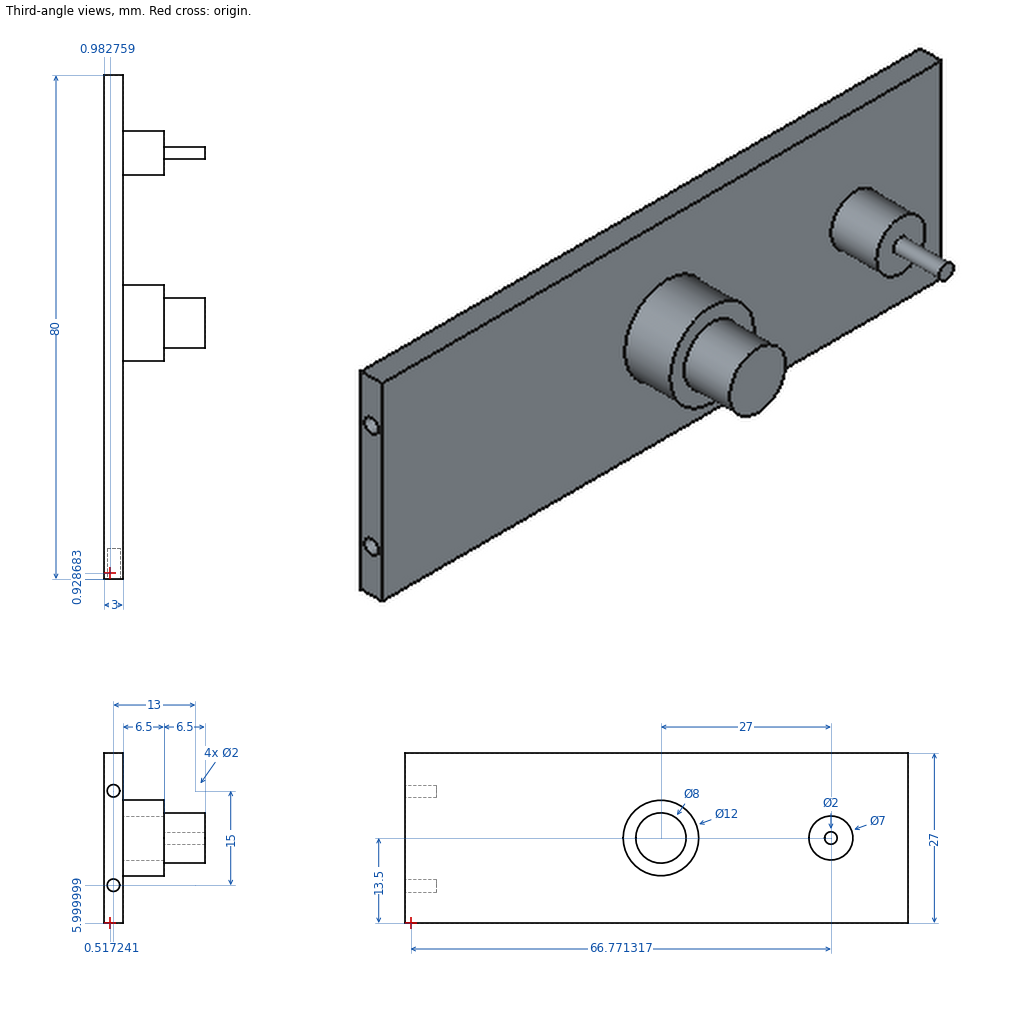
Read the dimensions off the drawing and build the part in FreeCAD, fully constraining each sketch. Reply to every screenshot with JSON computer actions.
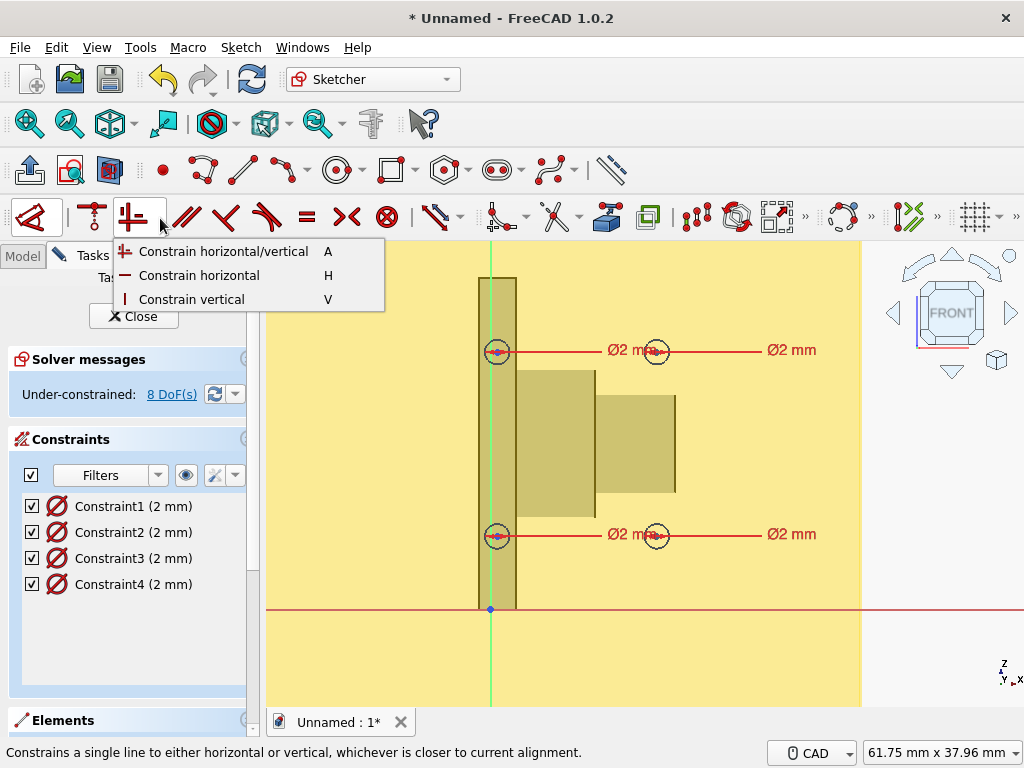
{"action": "left_click", "coordinate": [249, 299]}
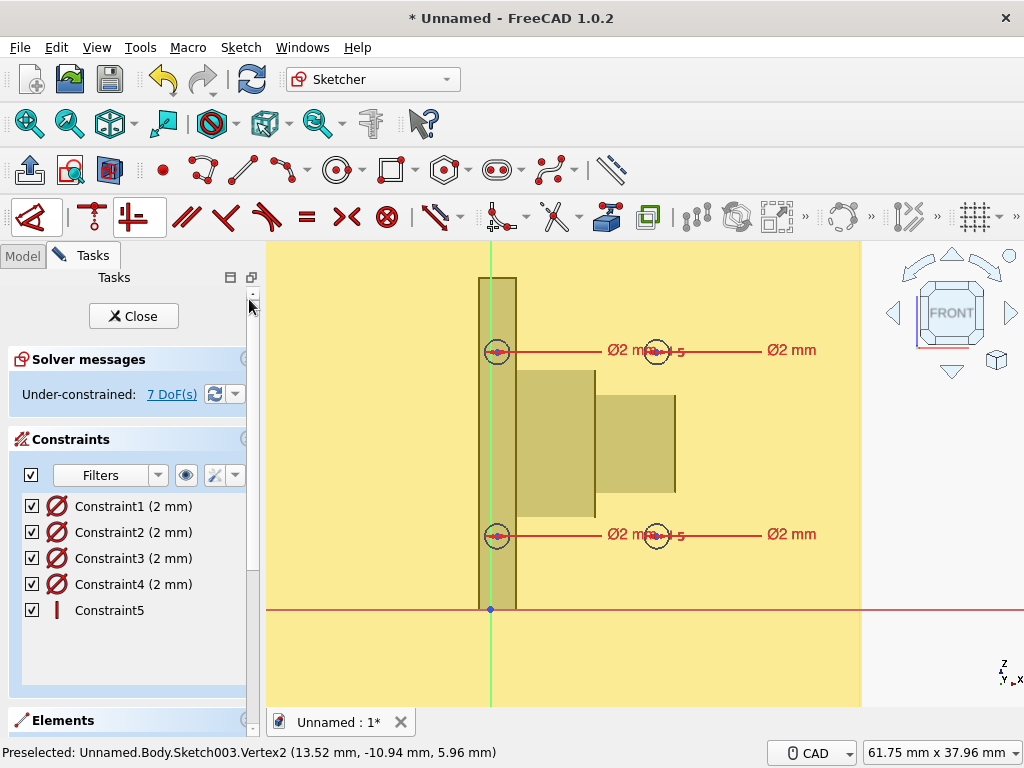
{"action": "left_click", "coordinate": [657, 352]}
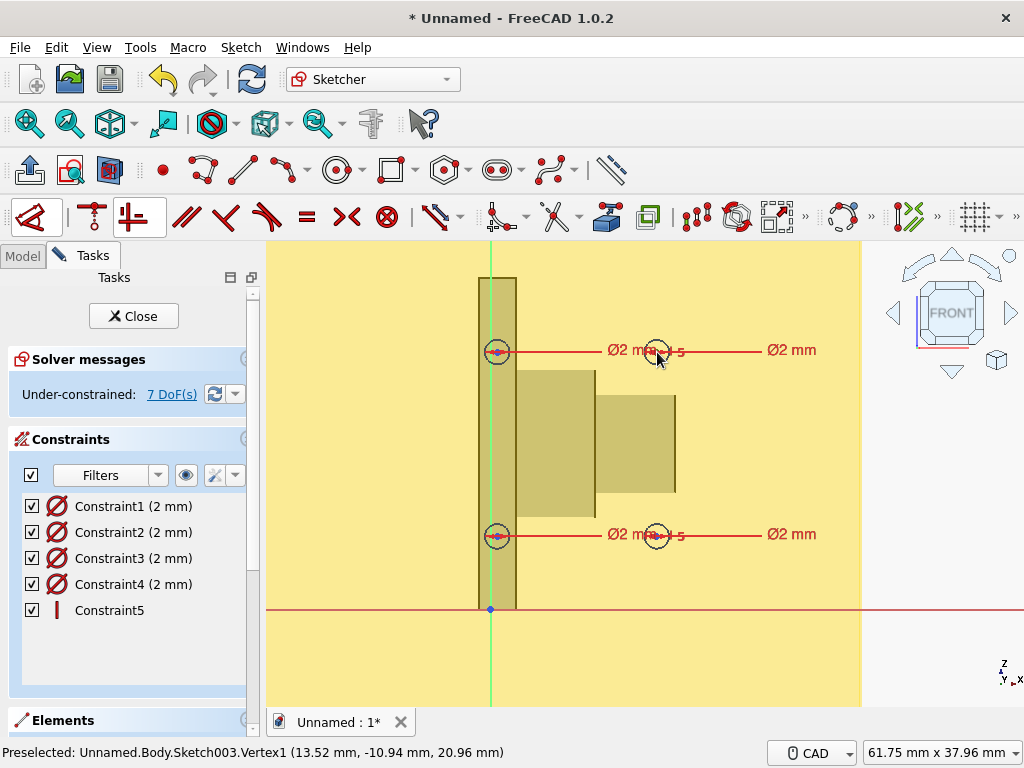
{"action": "left_click", "coordinate": [497, 352]}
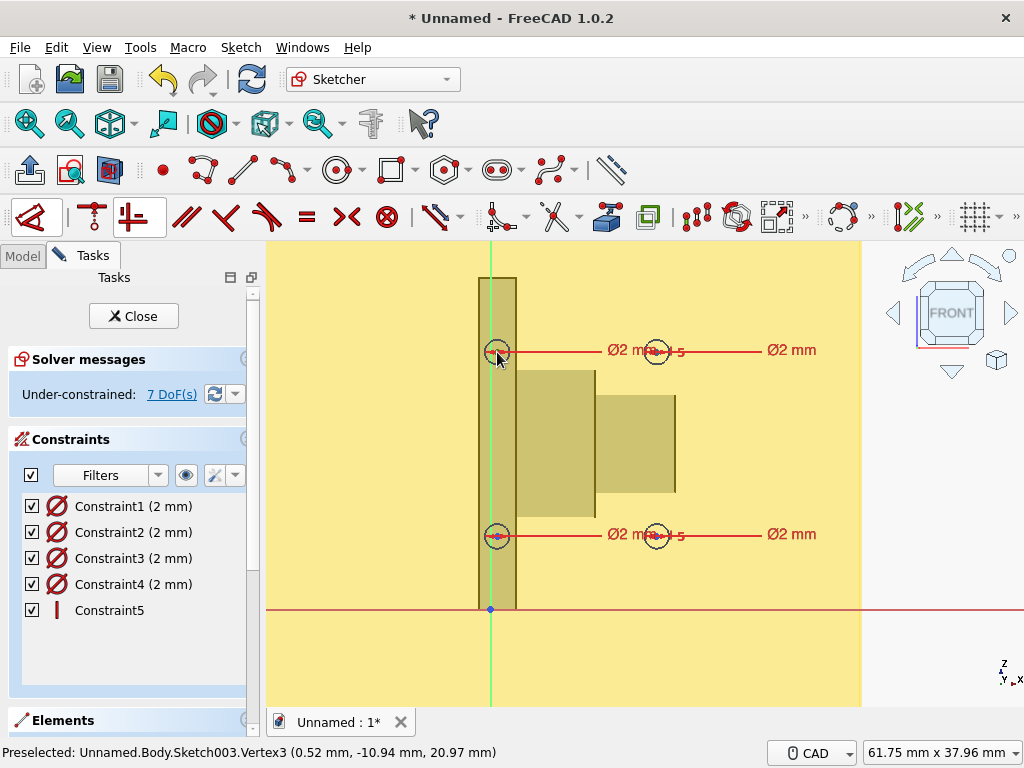
{"action": "left_click", "coordinate": [160, 218]}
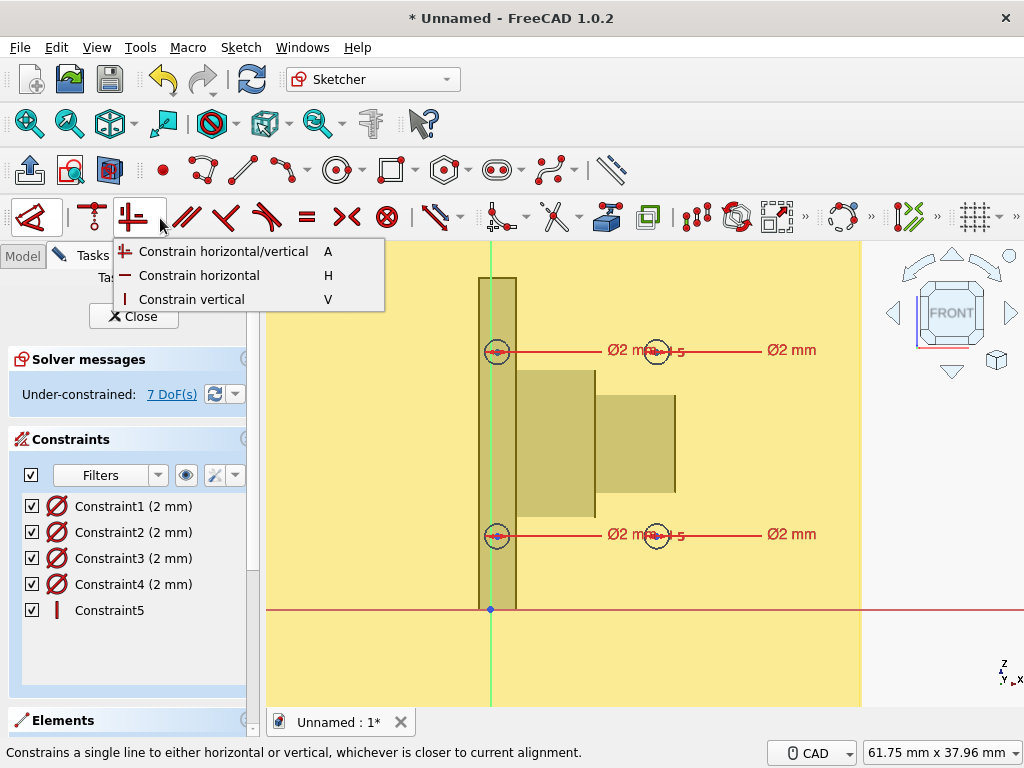
{"action": "left_click", "coordinate": [249, 275]}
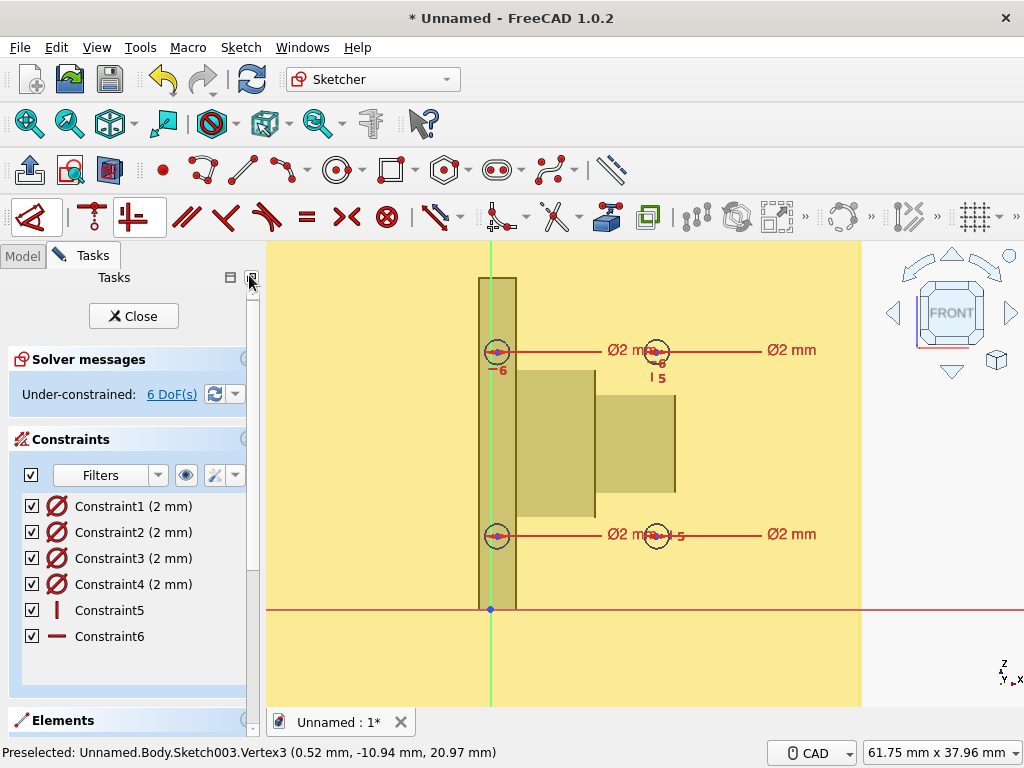
{"action": "left_click", "coordinate": [497, 352]}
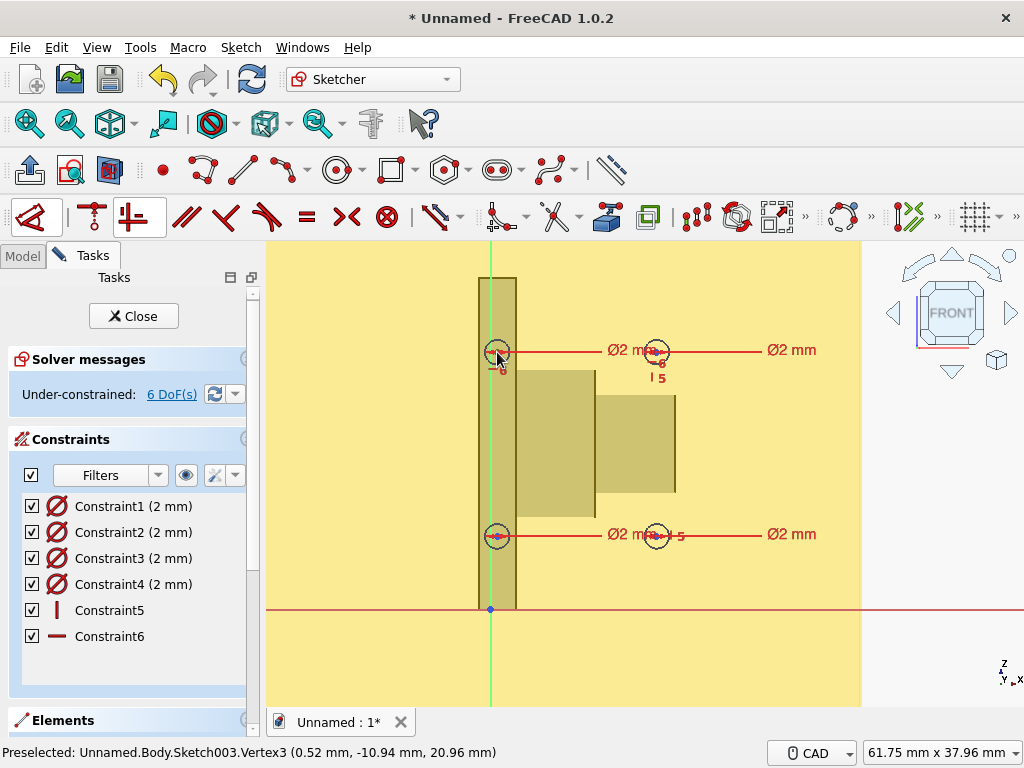
{"action": "left_click", "coordinate": [497, 536]}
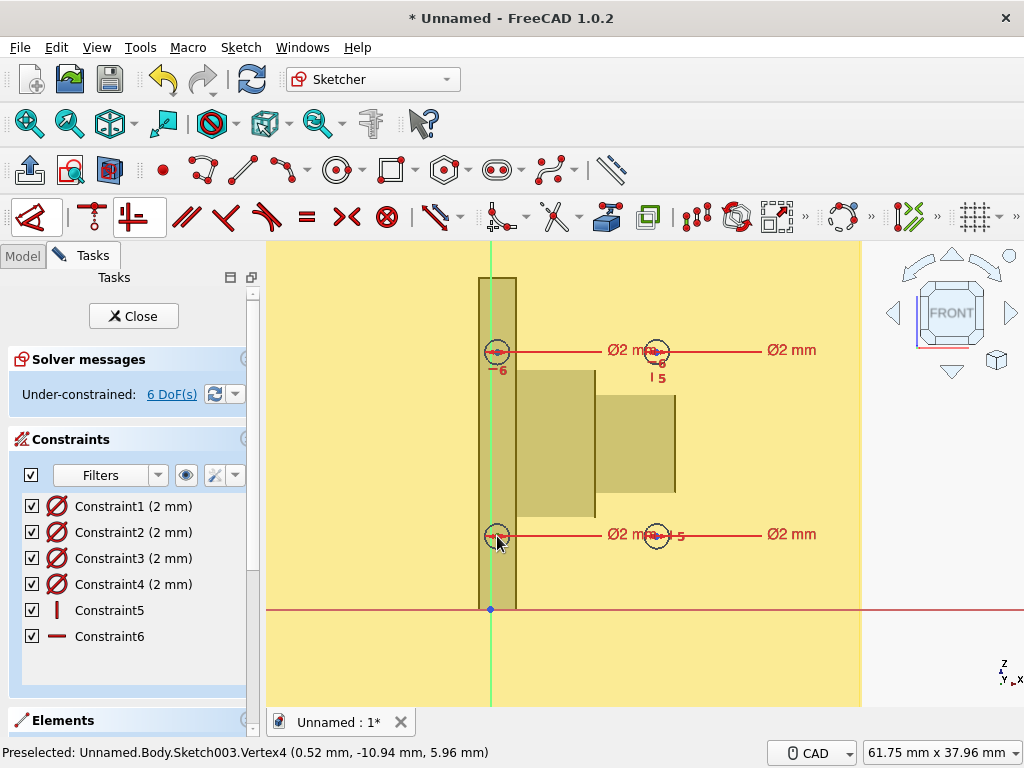
{"action": "left_click", "coordinate": [160, 218]}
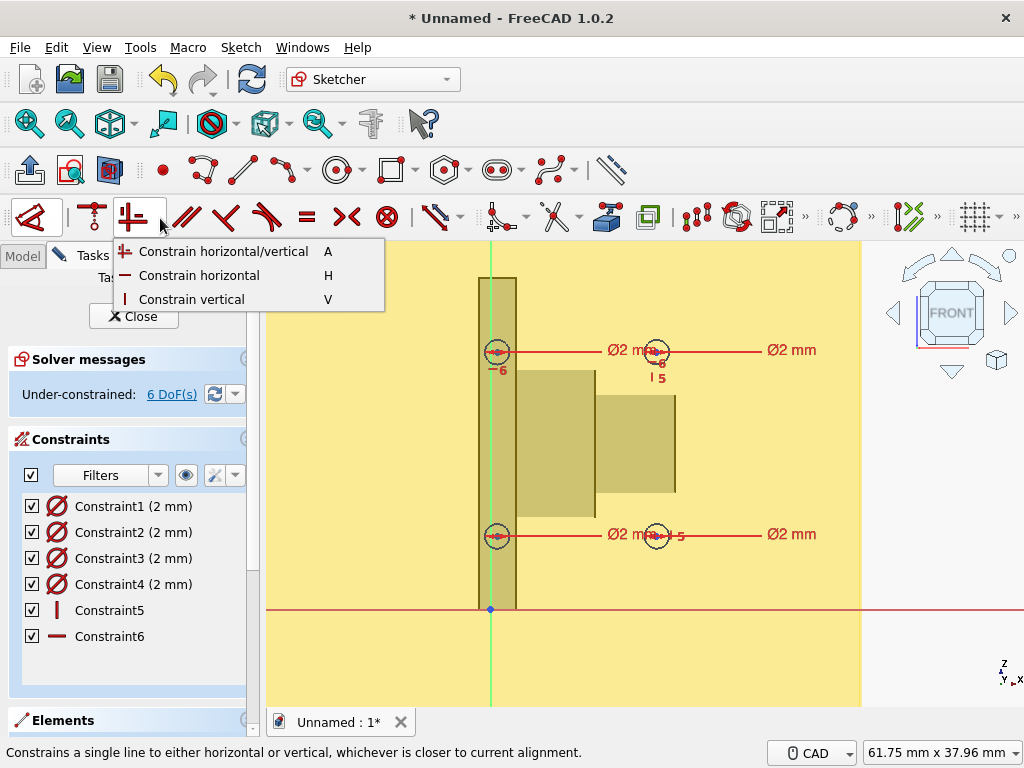
{"action": "left_click", "coordinate": [249, 299]}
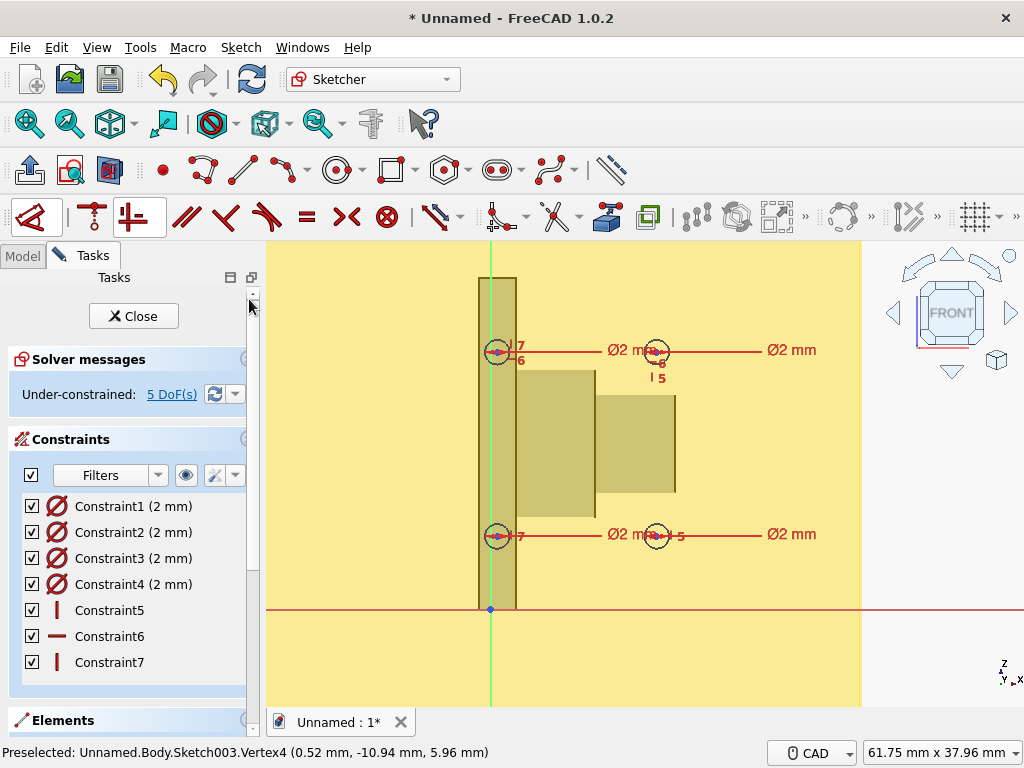
{"action": "left_click", "coordinate": [657, 536]}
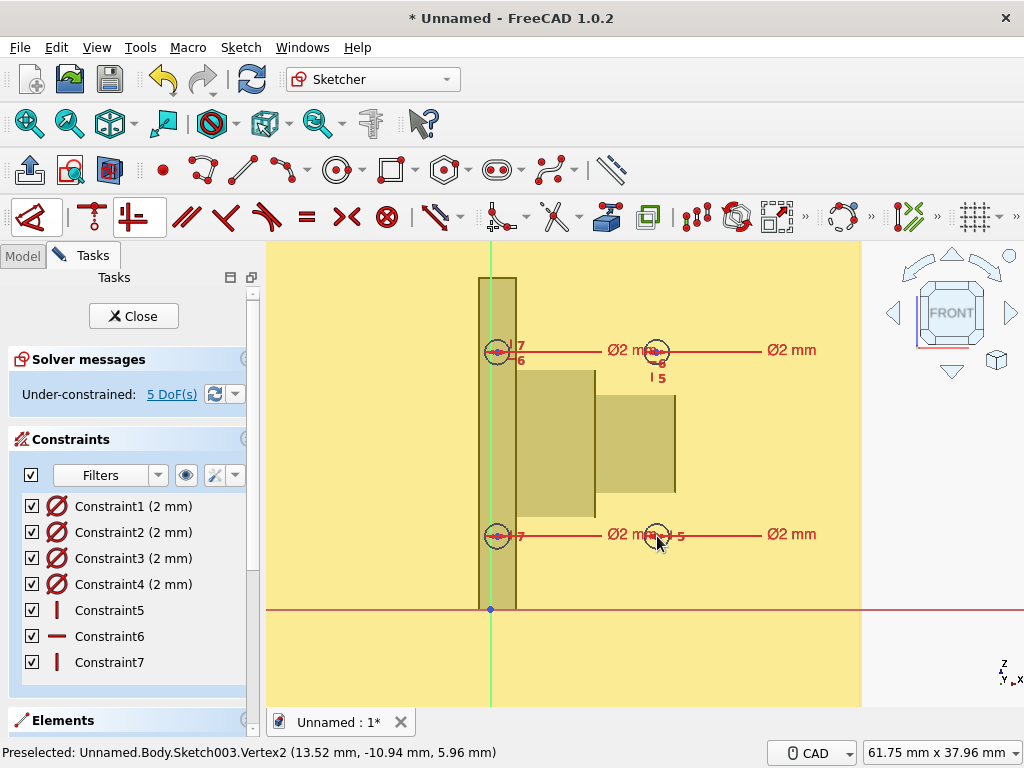
{"action": "left_click", "coordinate": [497, 536]}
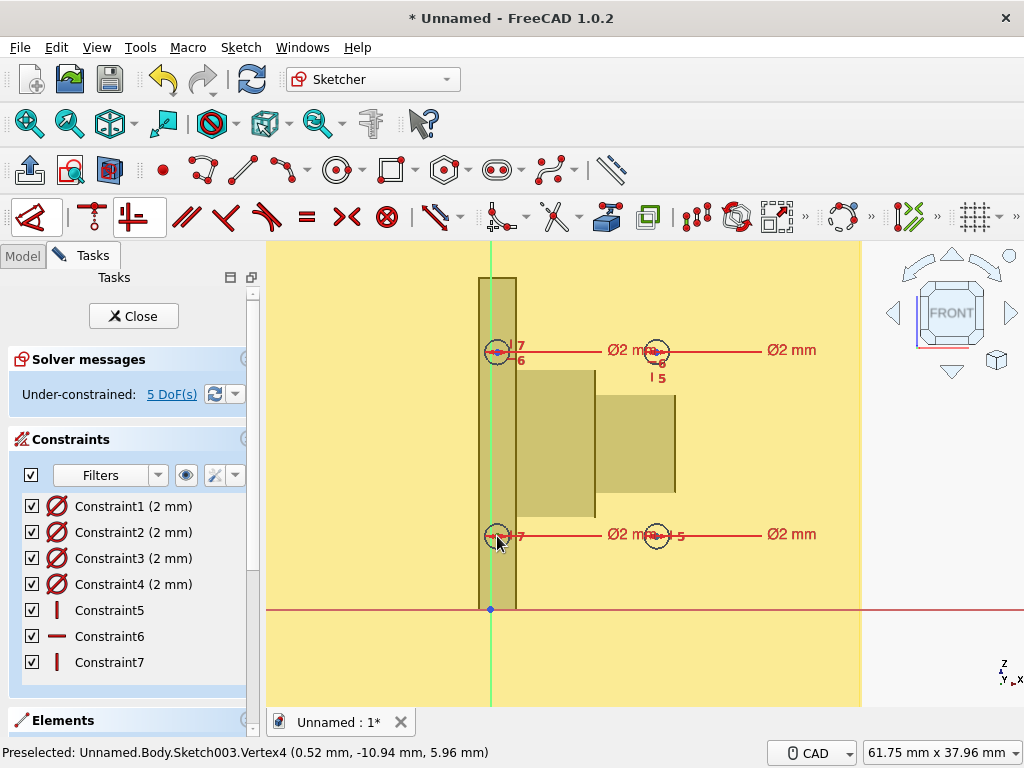
{"action": "key", "text": "h"}